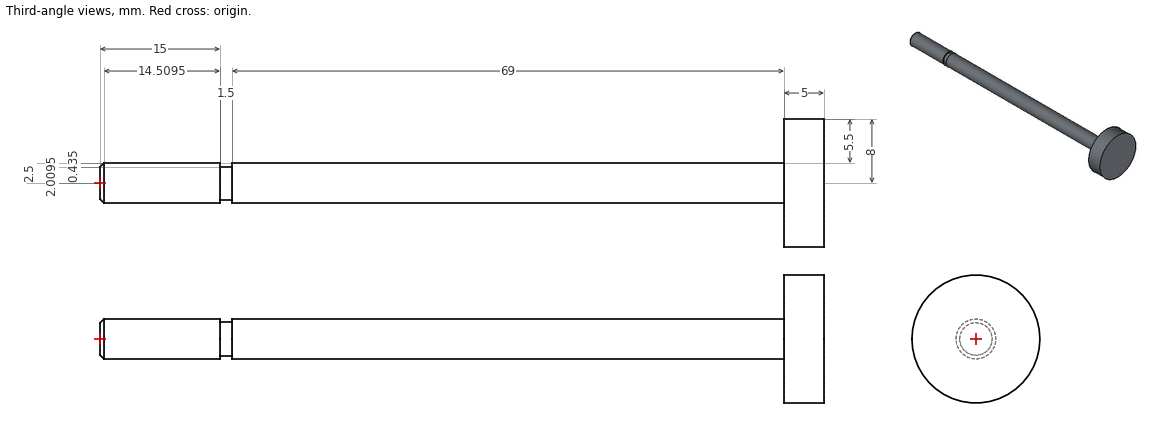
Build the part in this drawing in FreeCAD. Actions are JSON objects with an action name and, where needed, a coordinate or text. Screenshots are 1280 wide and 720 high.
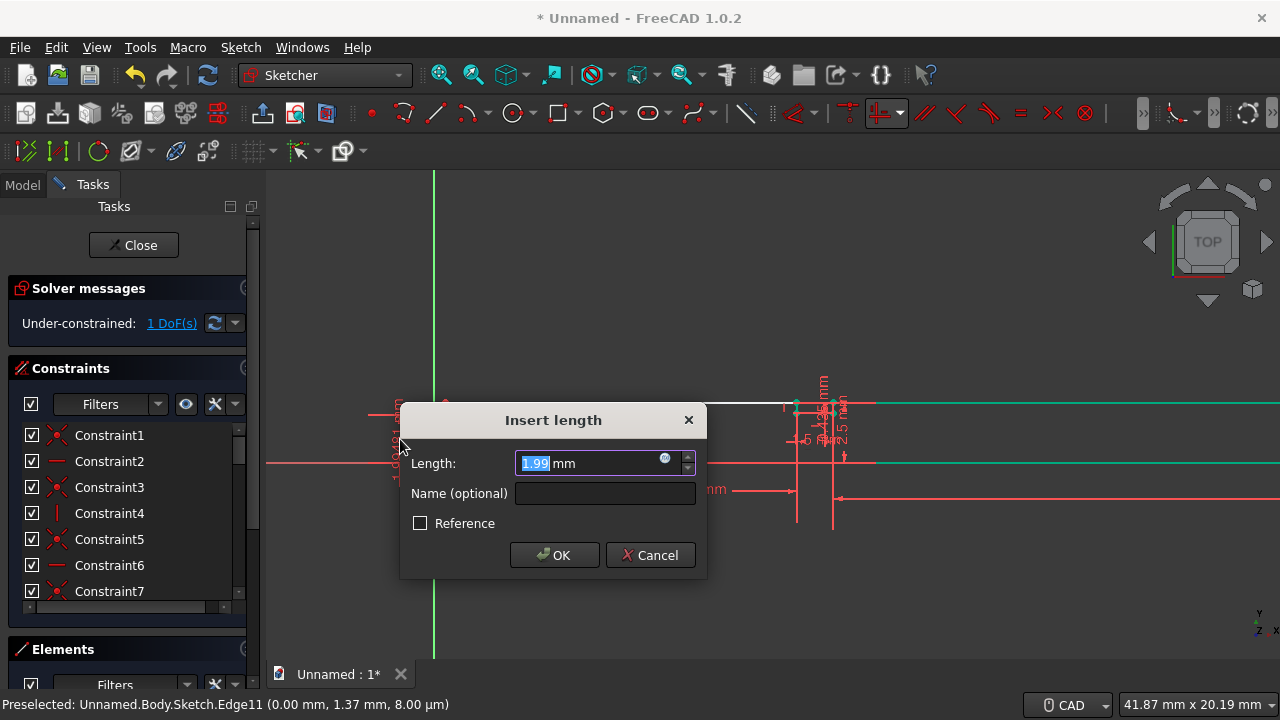
{"action": "type", "text": "2.0095"}
{"action": "key", "text": "Return"}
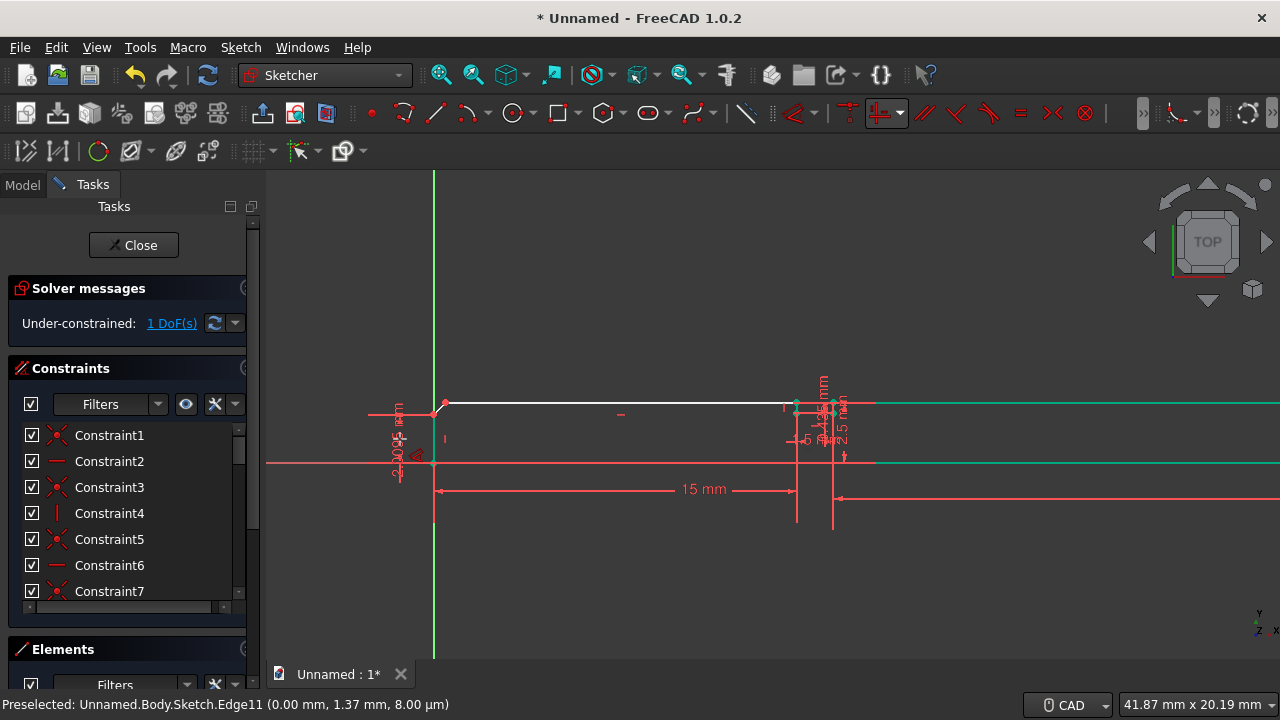
{"action": "scroll", "coordinate": [434, 430], "scroll_direction": "down", "scroll_amount": 7}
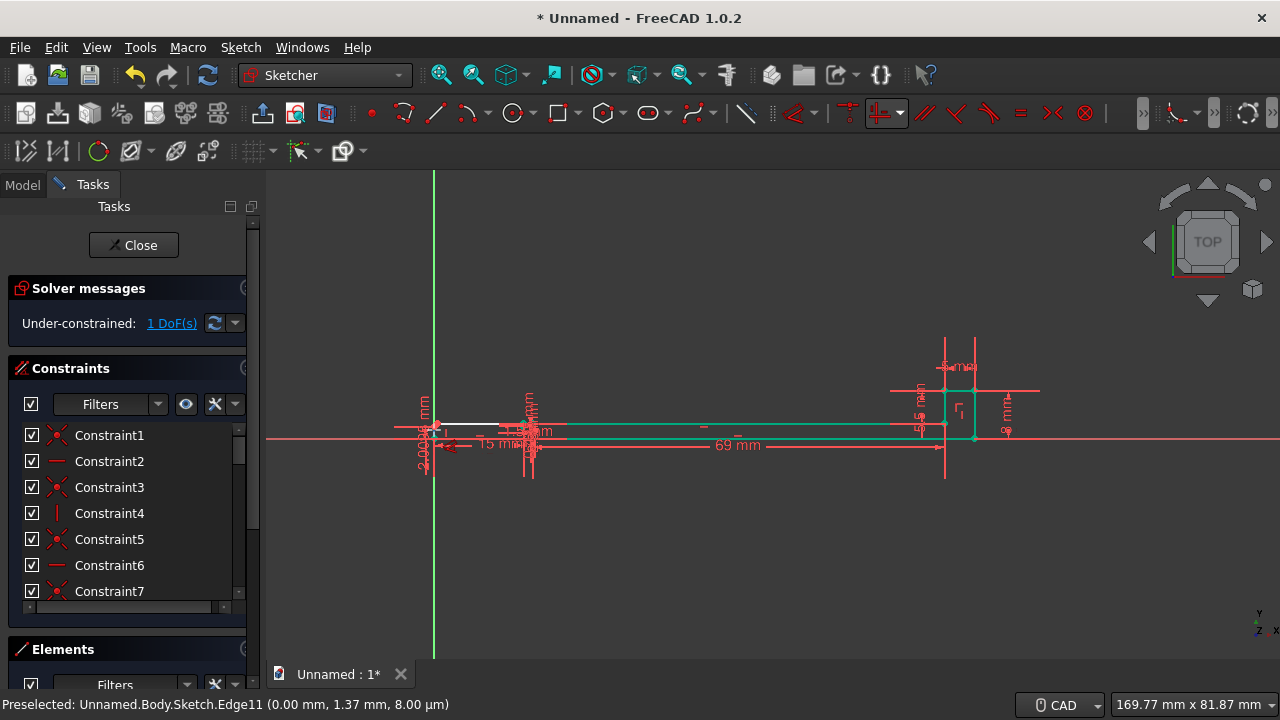
{"action": "left_click", "coordinate": [498, 424]}
{"action": "left_click", "coordinate": [480, 390]}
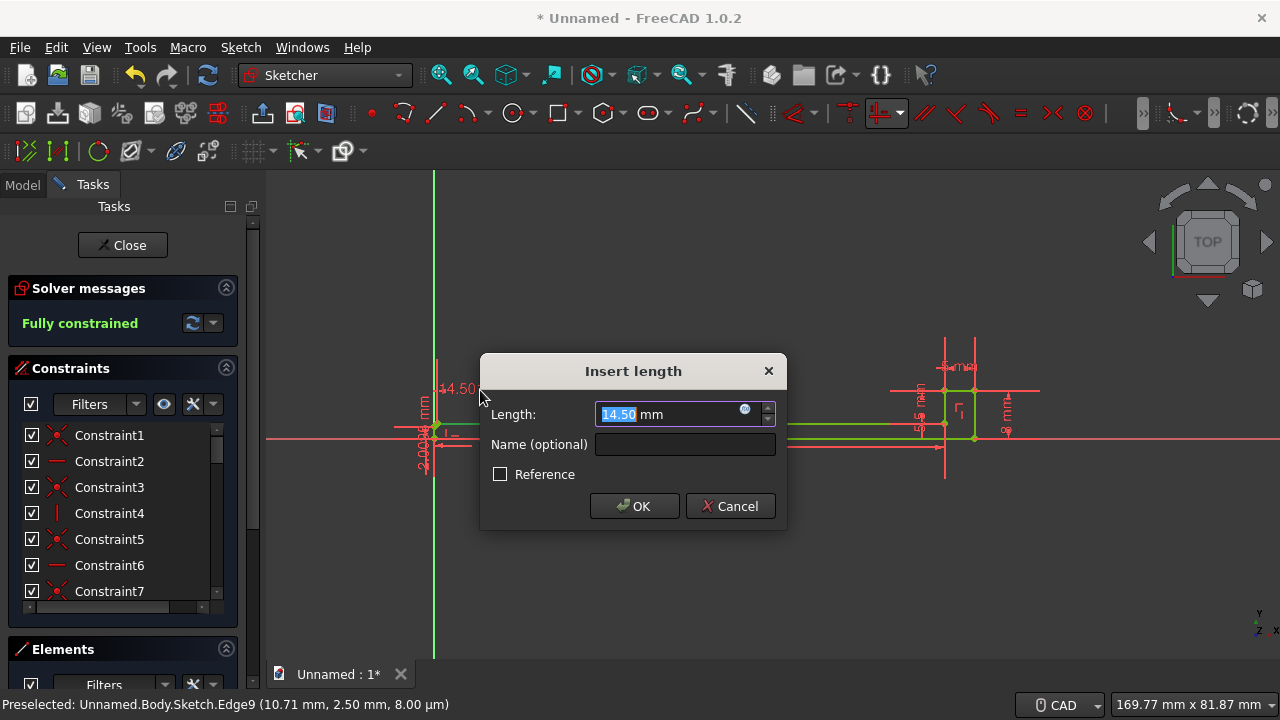
{"action": "type", "text": "14.5095"}
{"action": "key", "text": "Return"}
{"action": "key", "text": "Escape"}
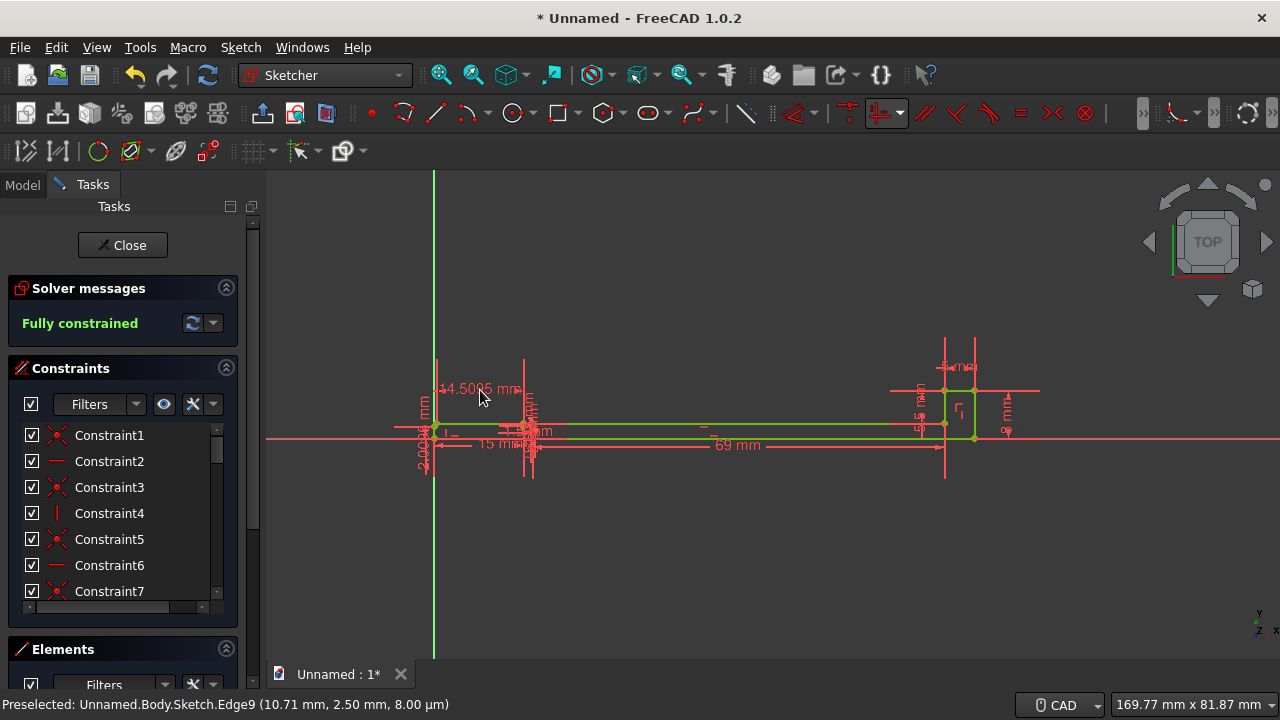
{"action": "left_click", "coordinate": [123, 245]}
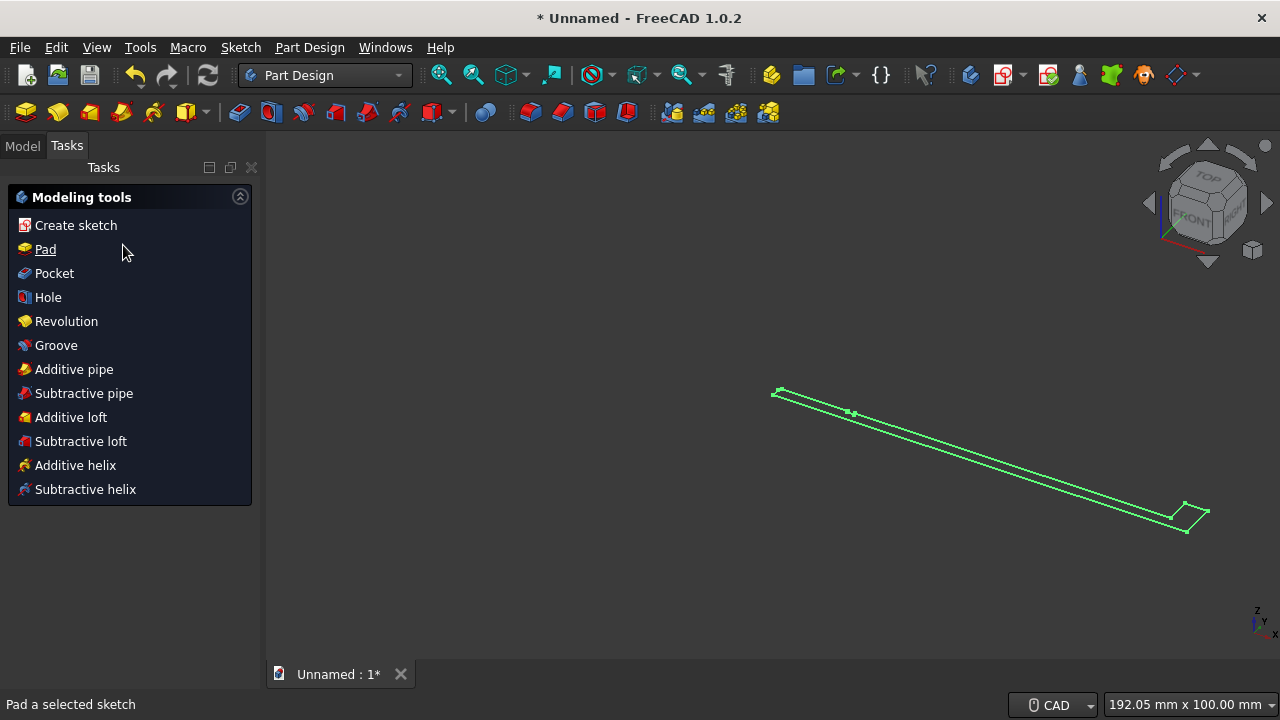
{"action": "left_click", "coordinate": [58, 112]}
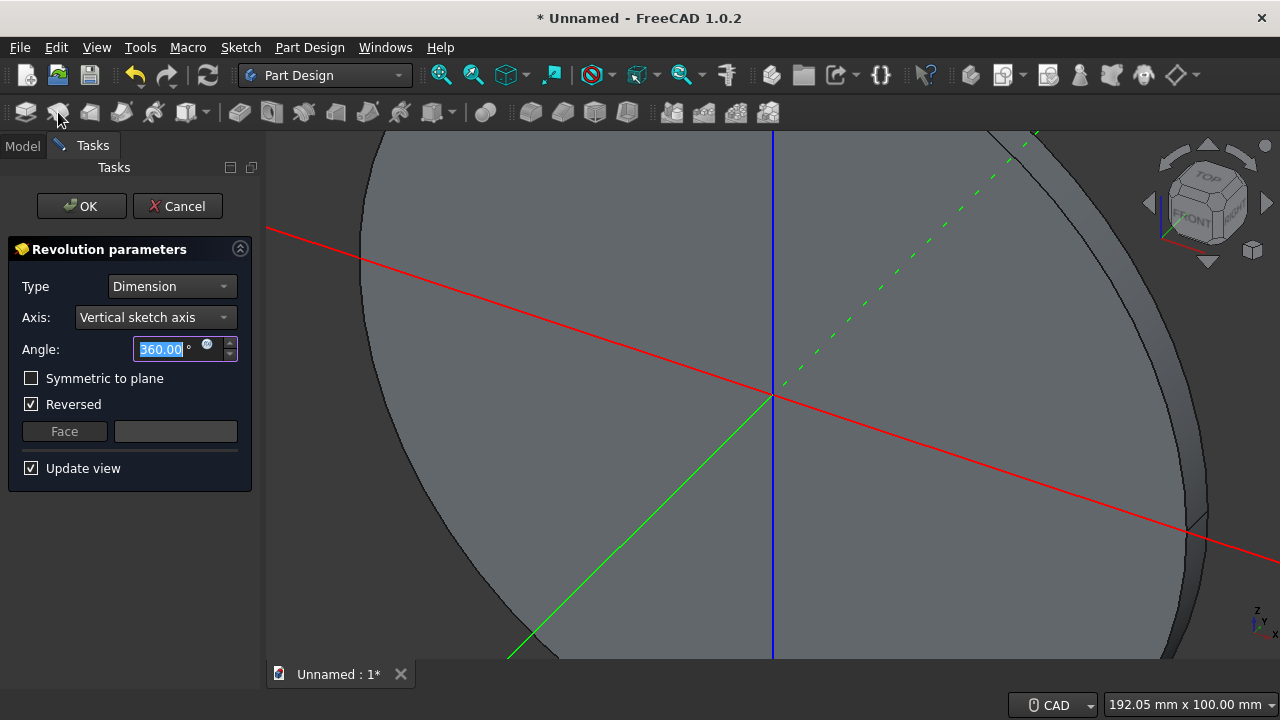
{"action": "left_click", "coordinate": [156, 318]}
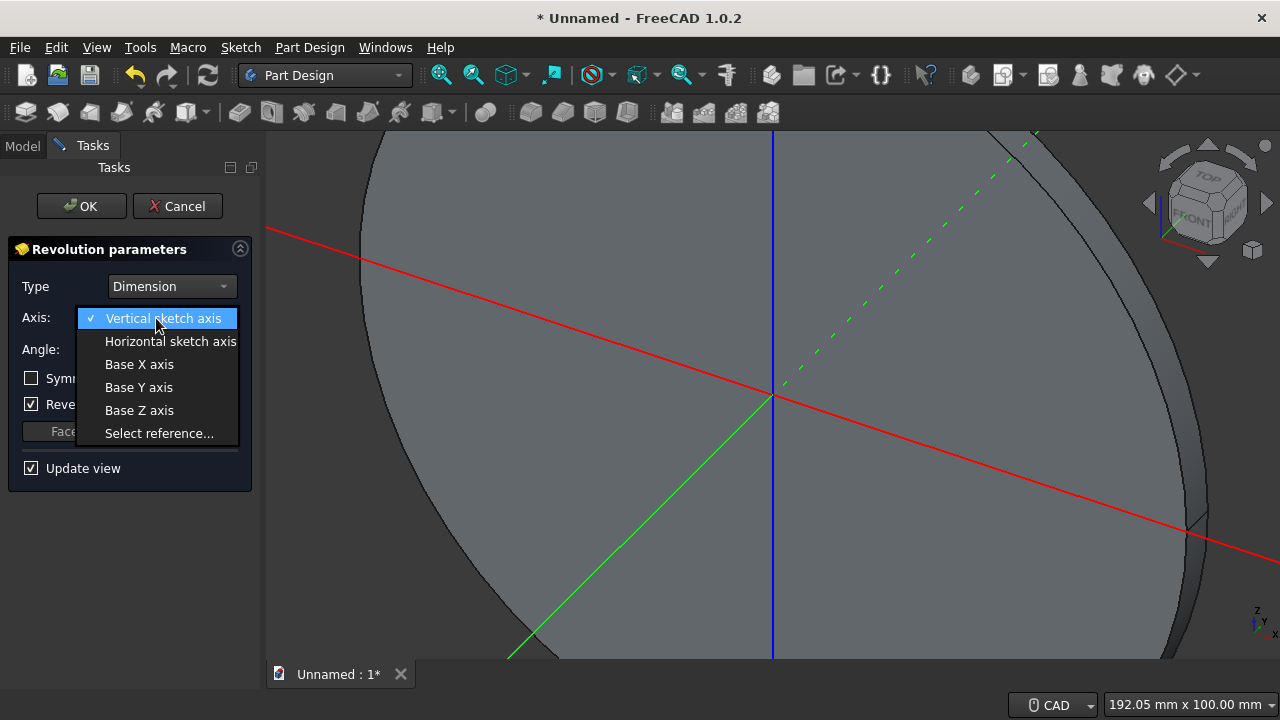
{"action": "left_click", "coordinate": [156, 342]}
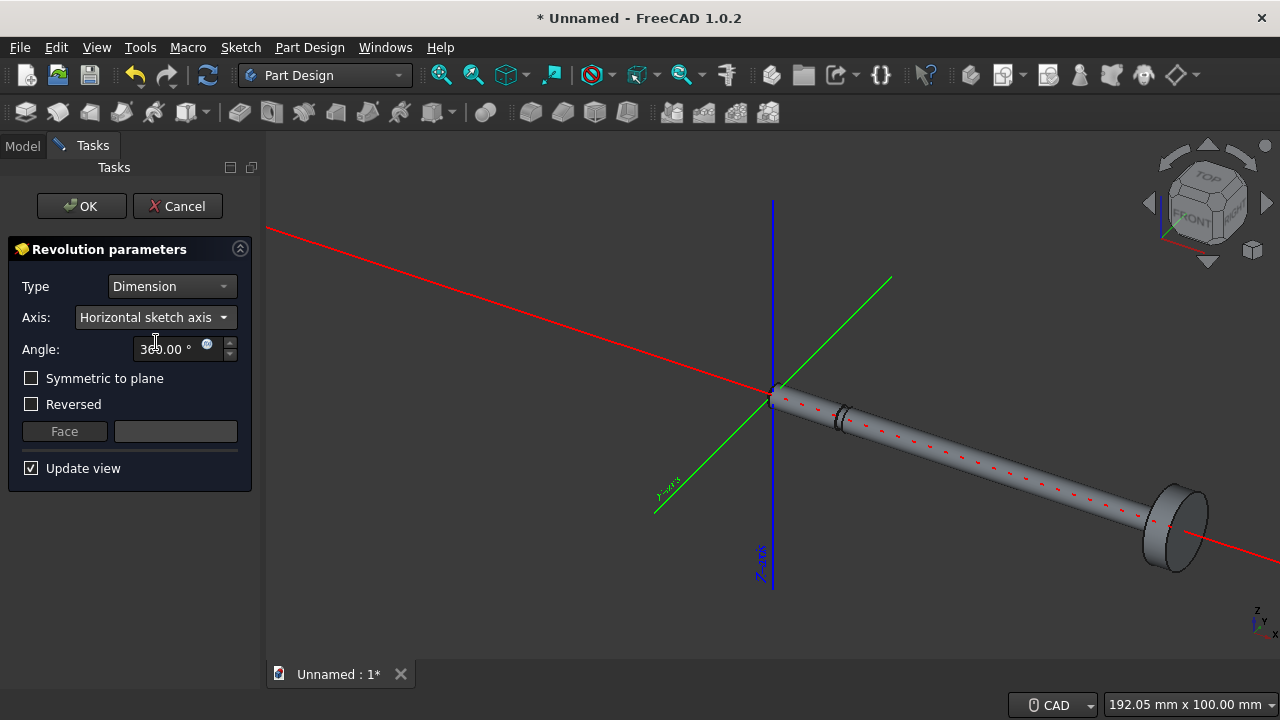
{"action": "left_click", "coordinate": [82, 206]}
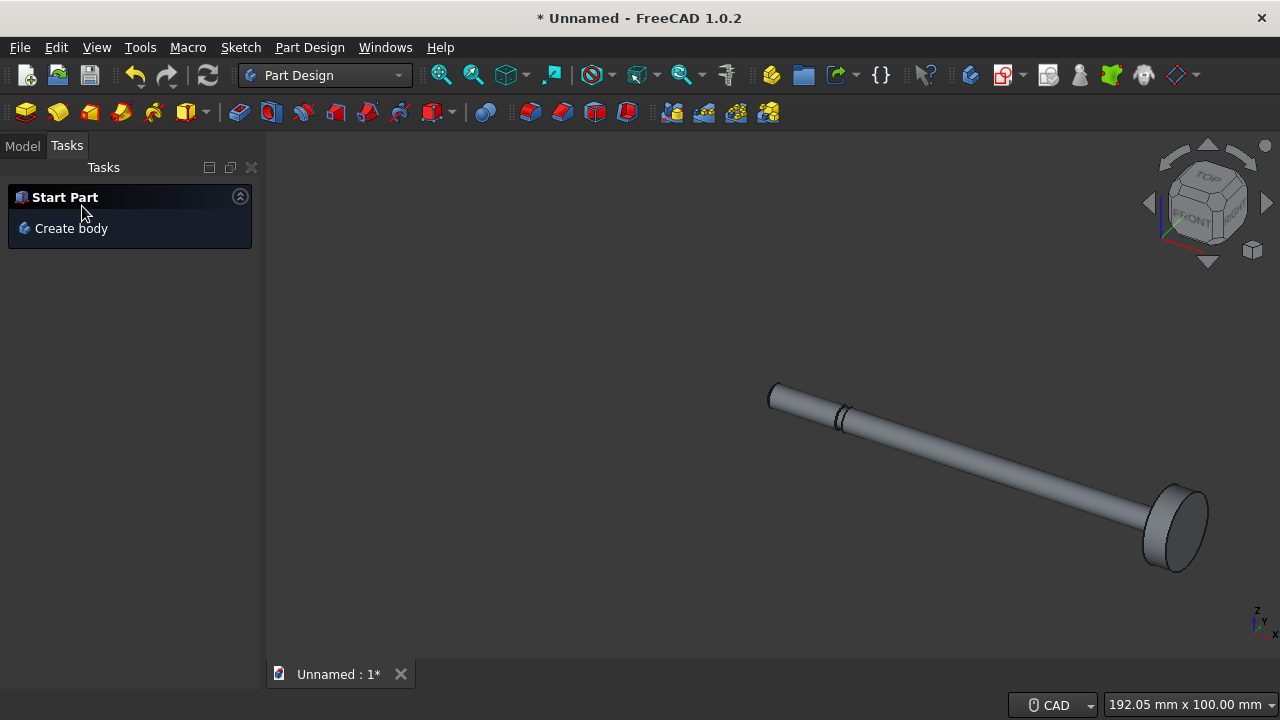
{"action": "key", "text": "0"}